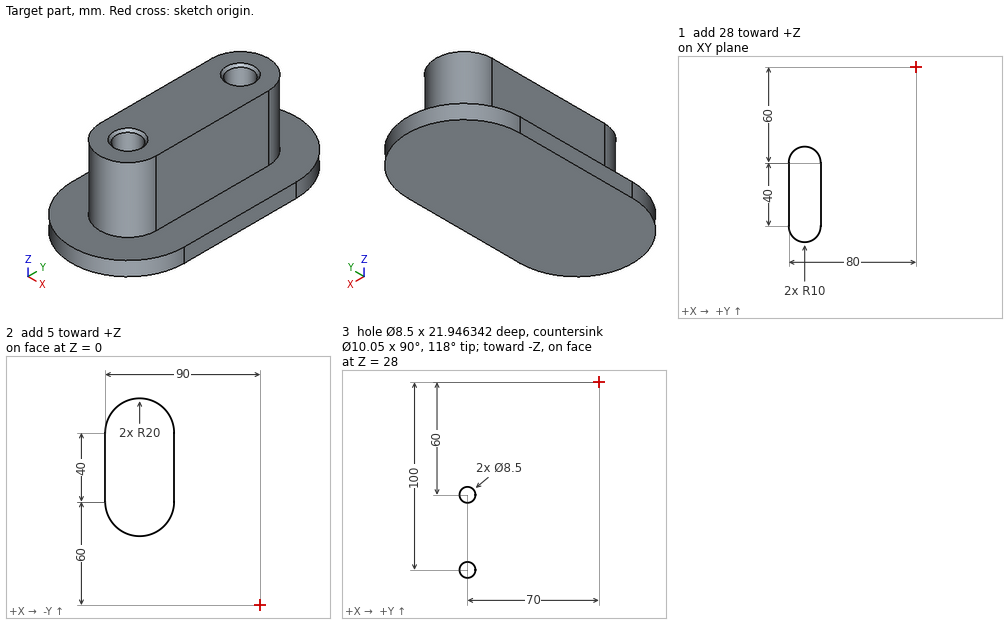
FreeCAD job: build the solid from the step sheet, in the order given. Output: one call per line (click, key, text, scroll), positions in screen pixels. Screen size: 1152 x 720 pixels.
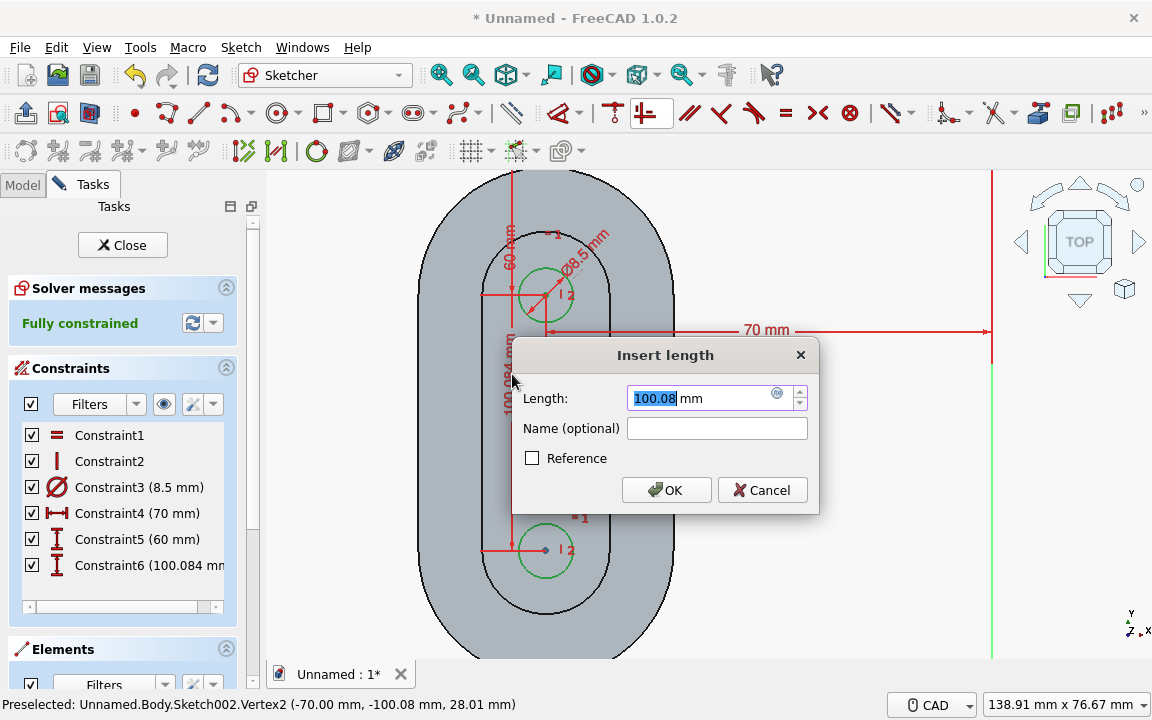
text(100)
key(Return)
key(Escape)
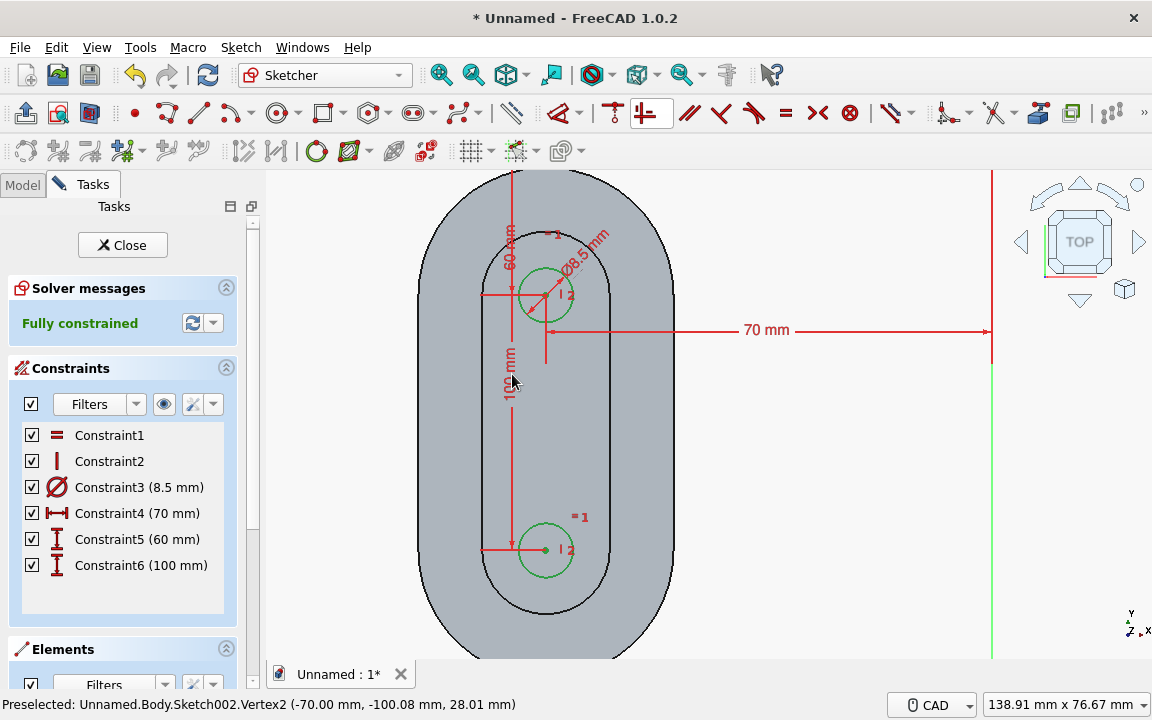
click(123, 245)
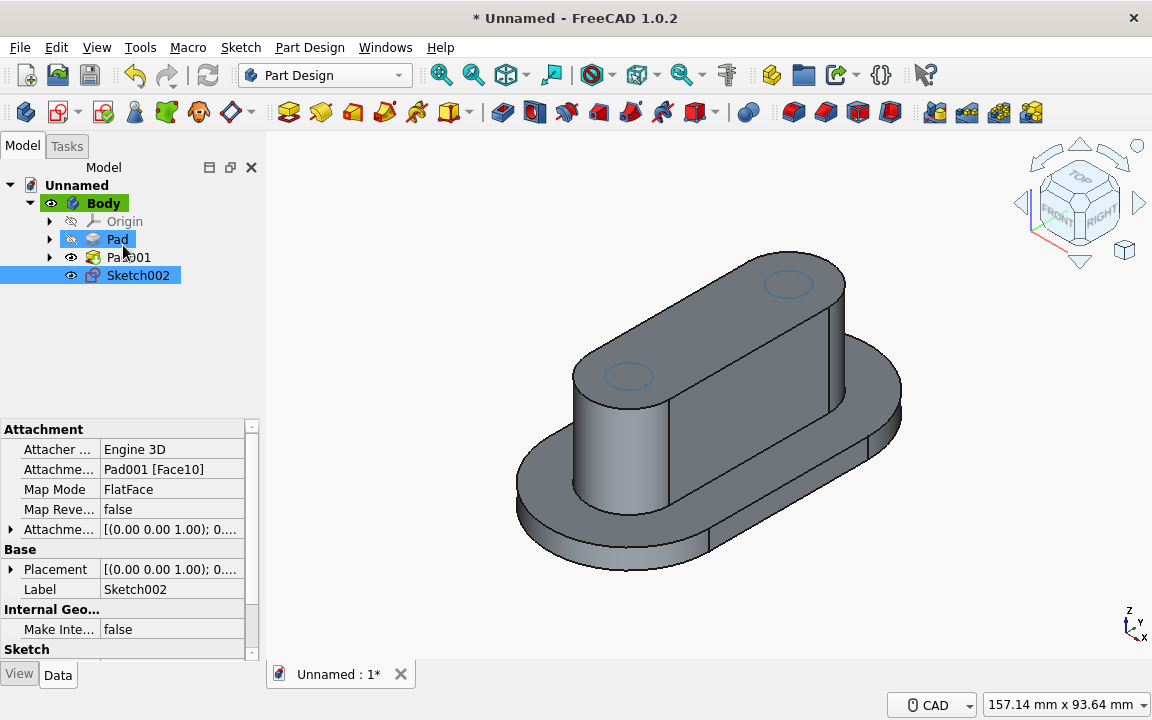
click(536, 112)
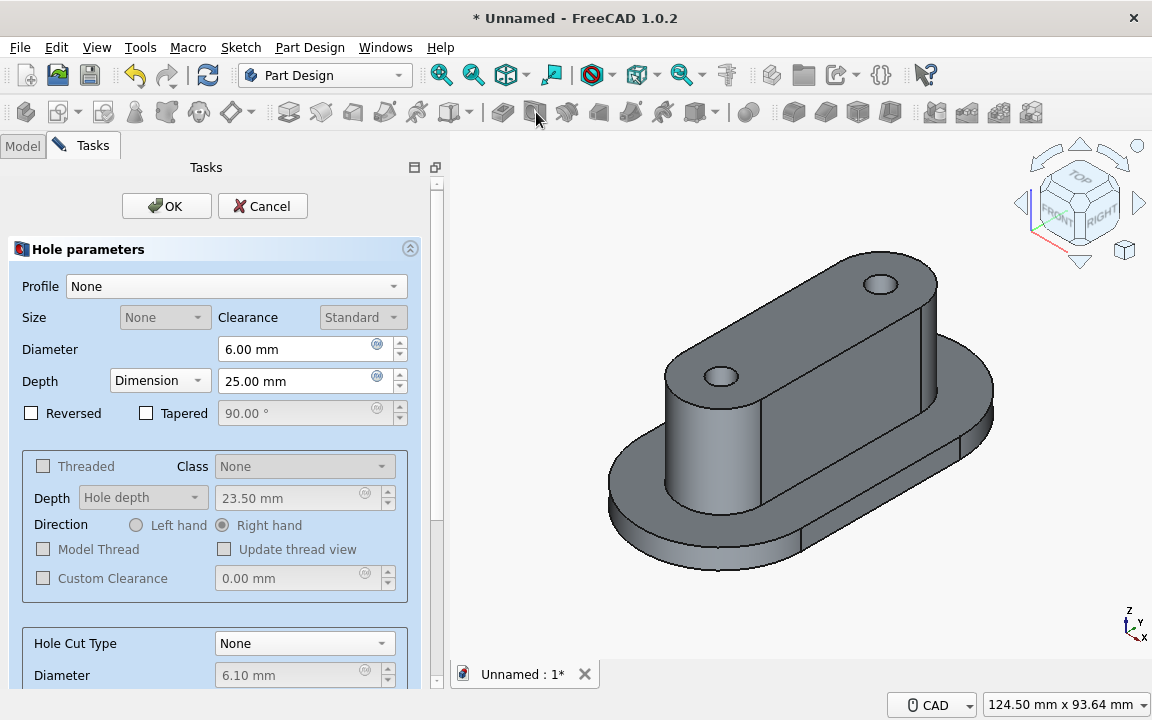
triple_click(305, 349)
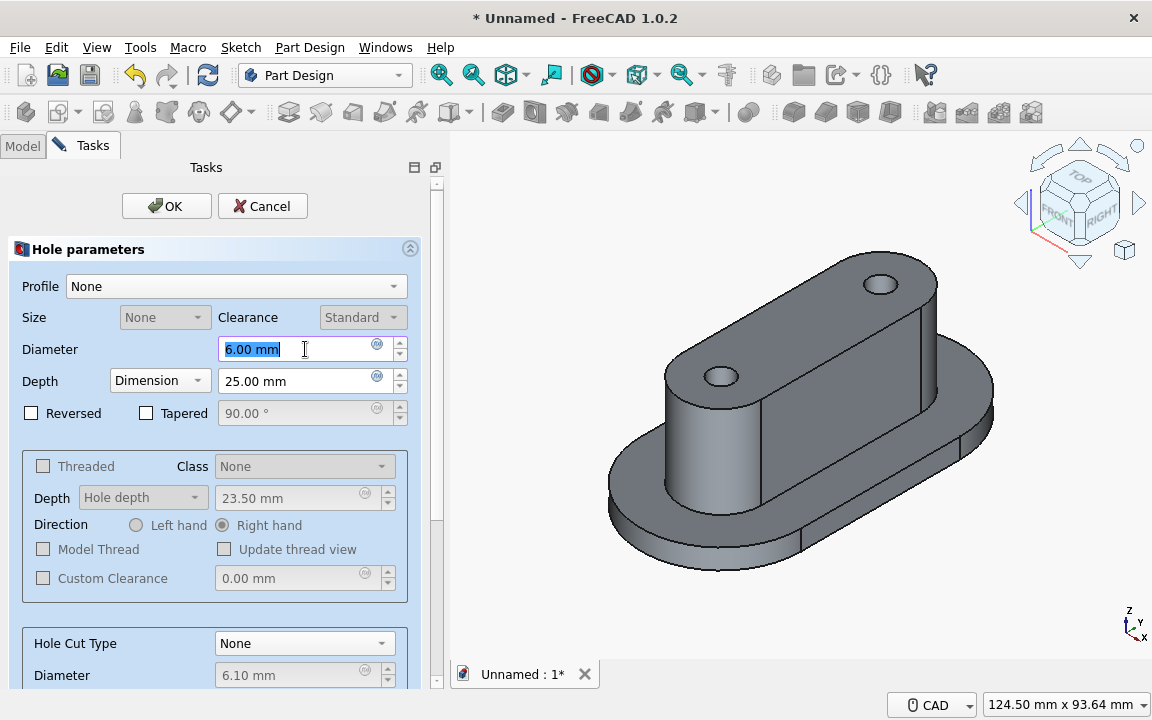
text(8.5)
key(Tab)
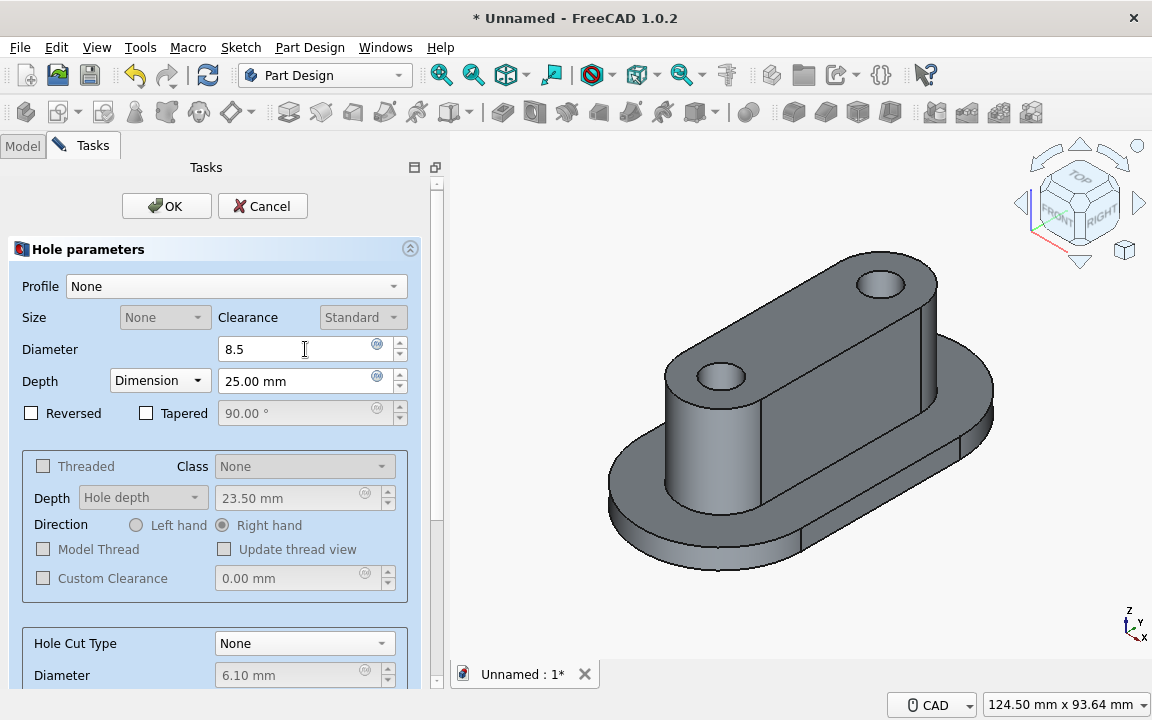
triple_click(305, 381)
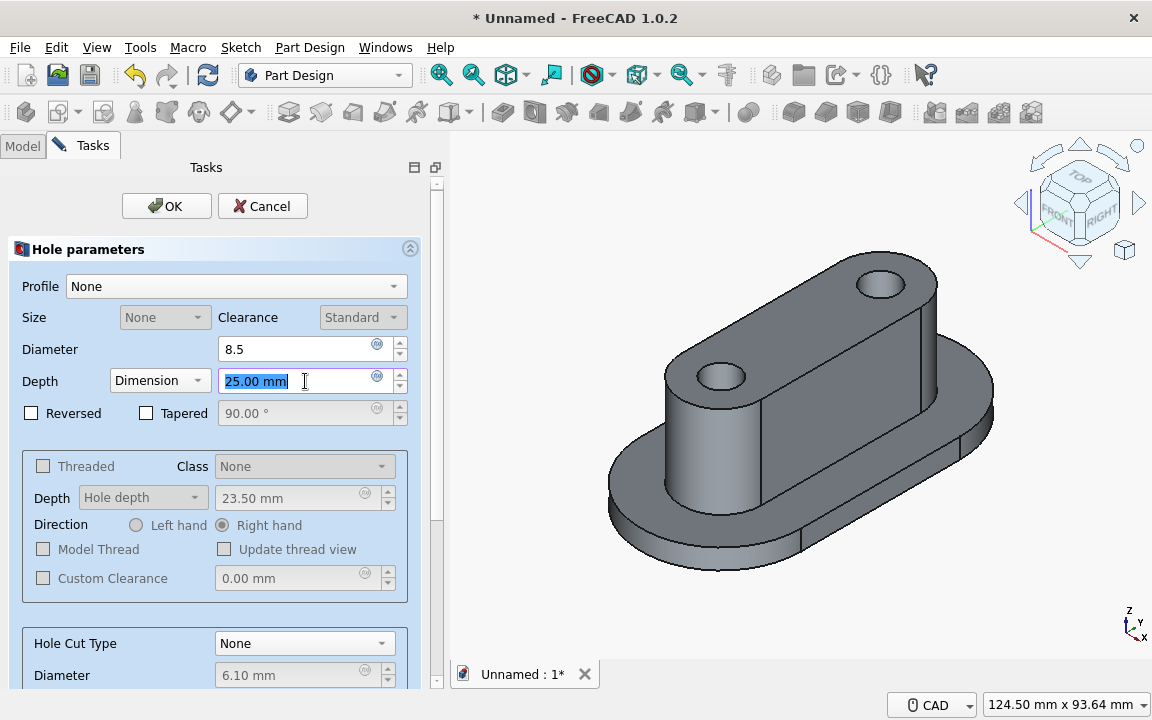
text(21.946342)
key(Tab)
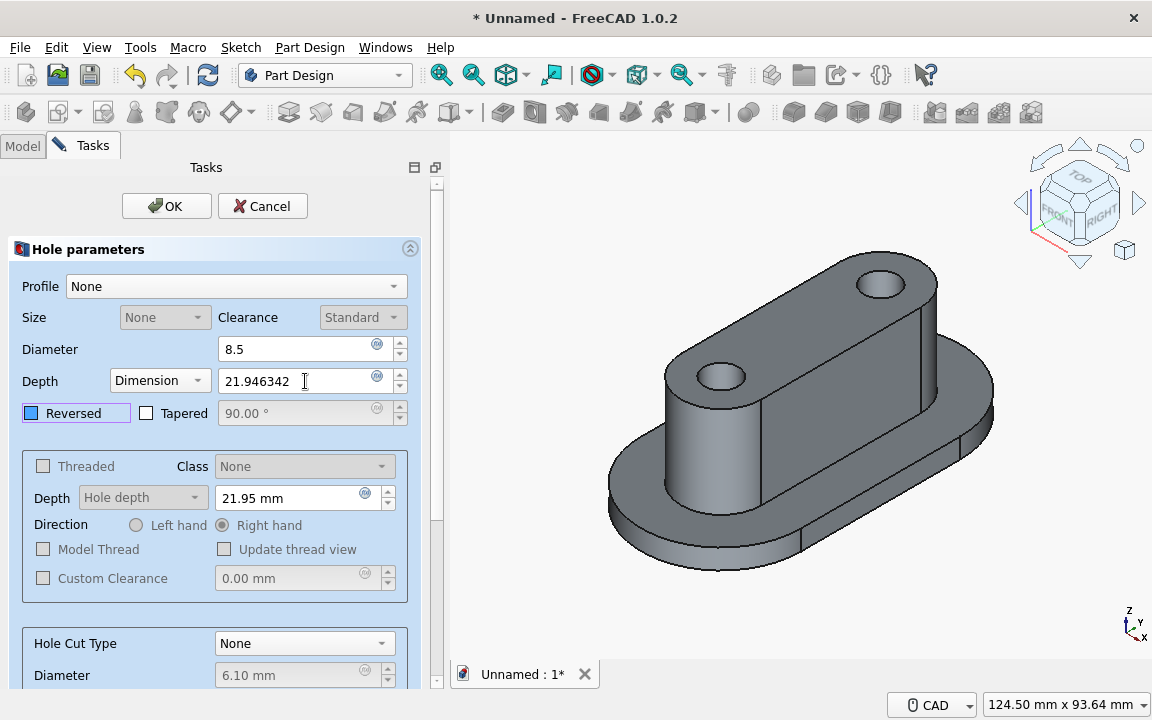
click(306, 644)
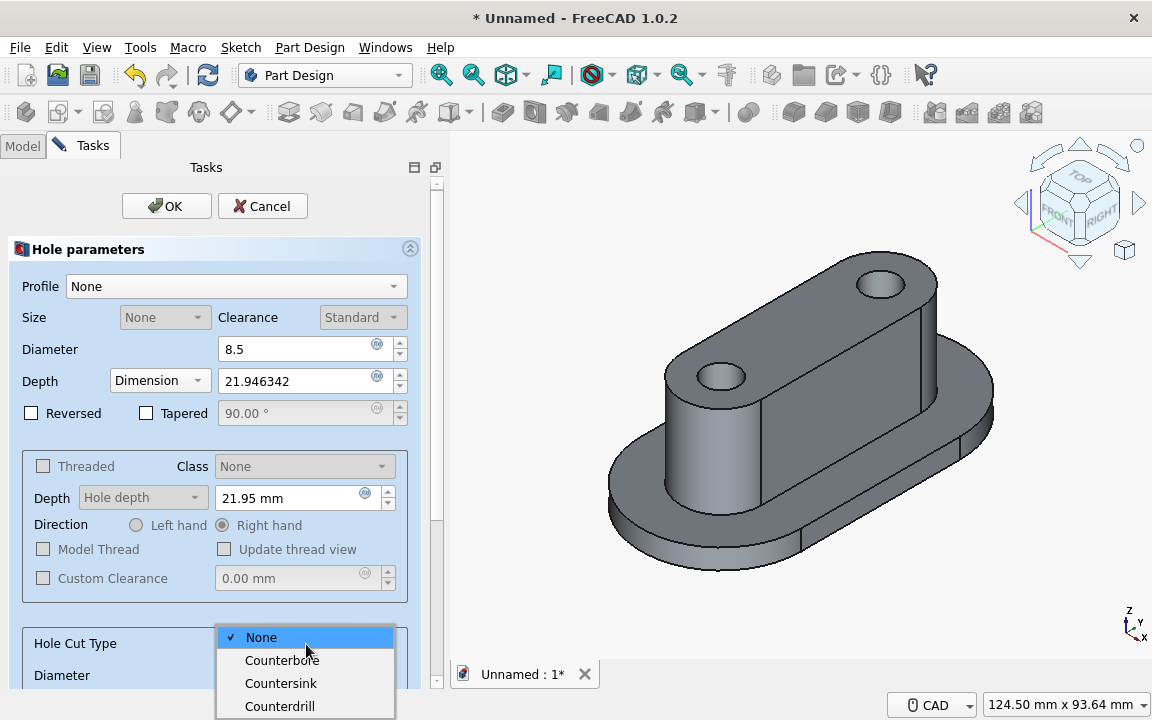
click(304, 684)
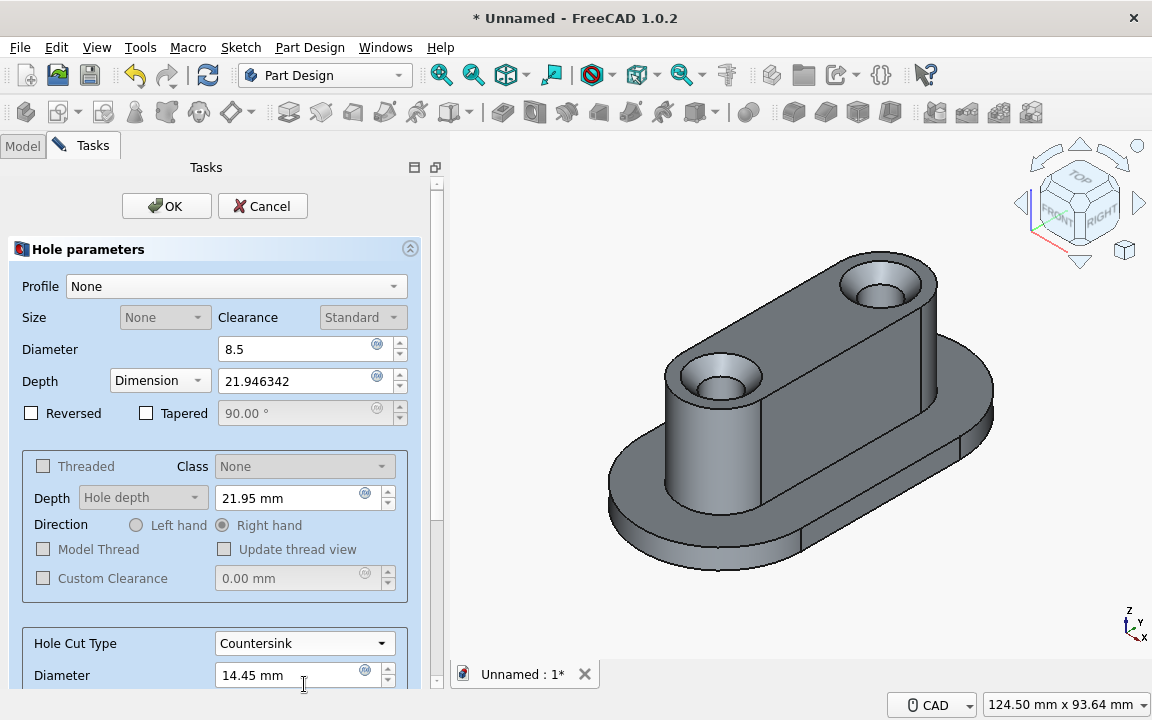
triple_click(298, 675)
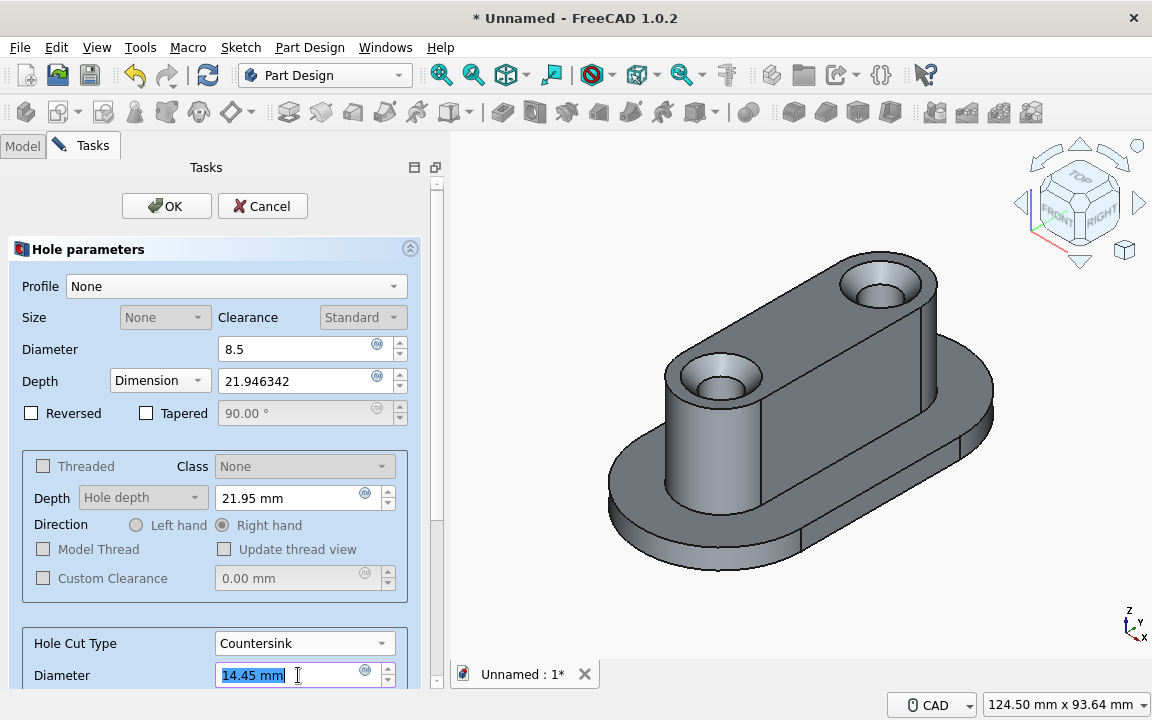
text(10.05)
key(Tab)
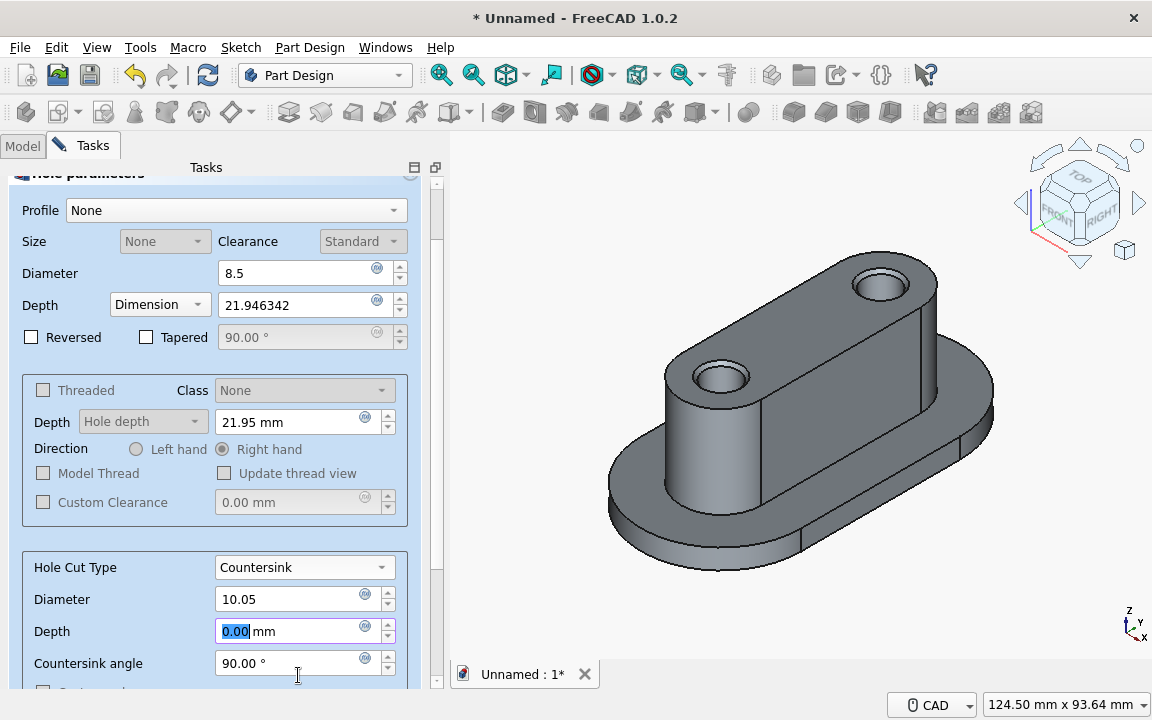
scroll(437, 432, up, 3)